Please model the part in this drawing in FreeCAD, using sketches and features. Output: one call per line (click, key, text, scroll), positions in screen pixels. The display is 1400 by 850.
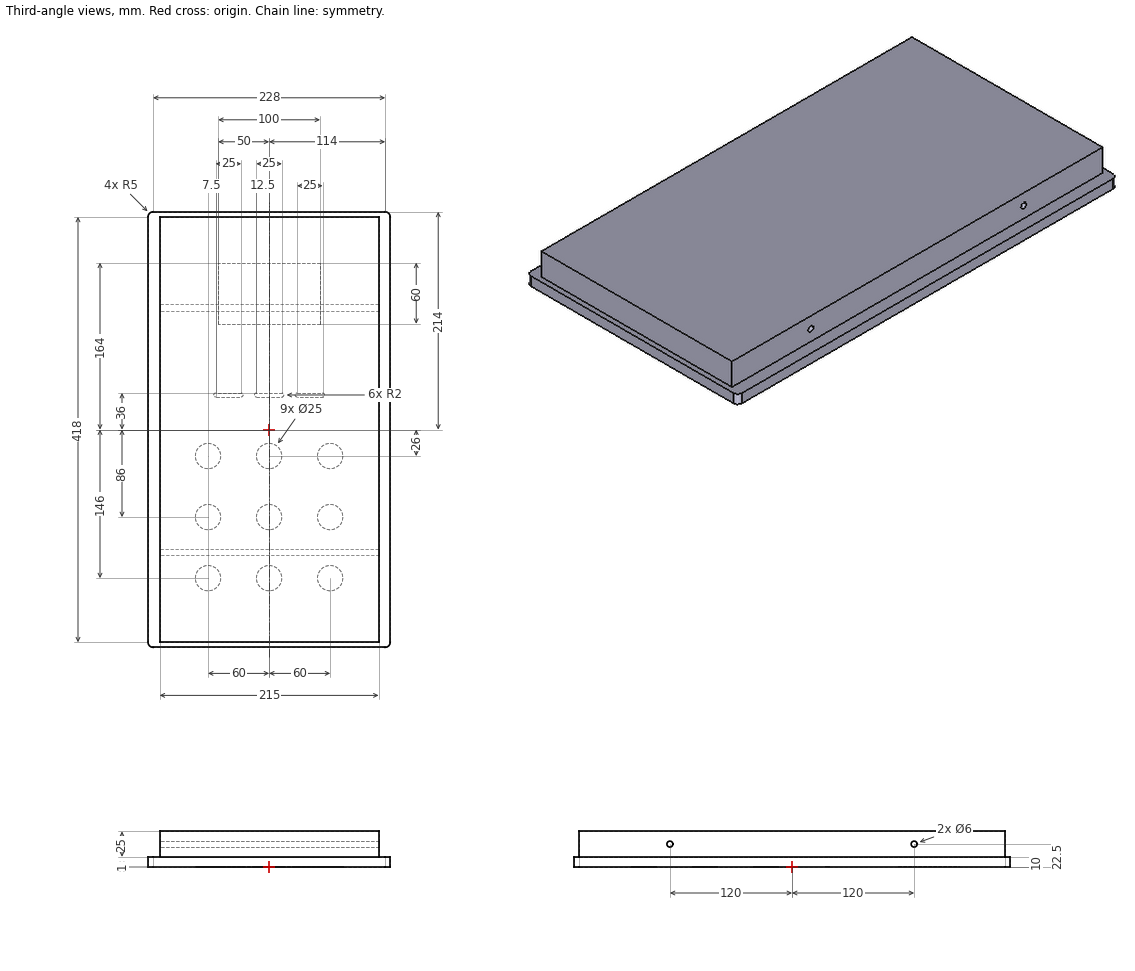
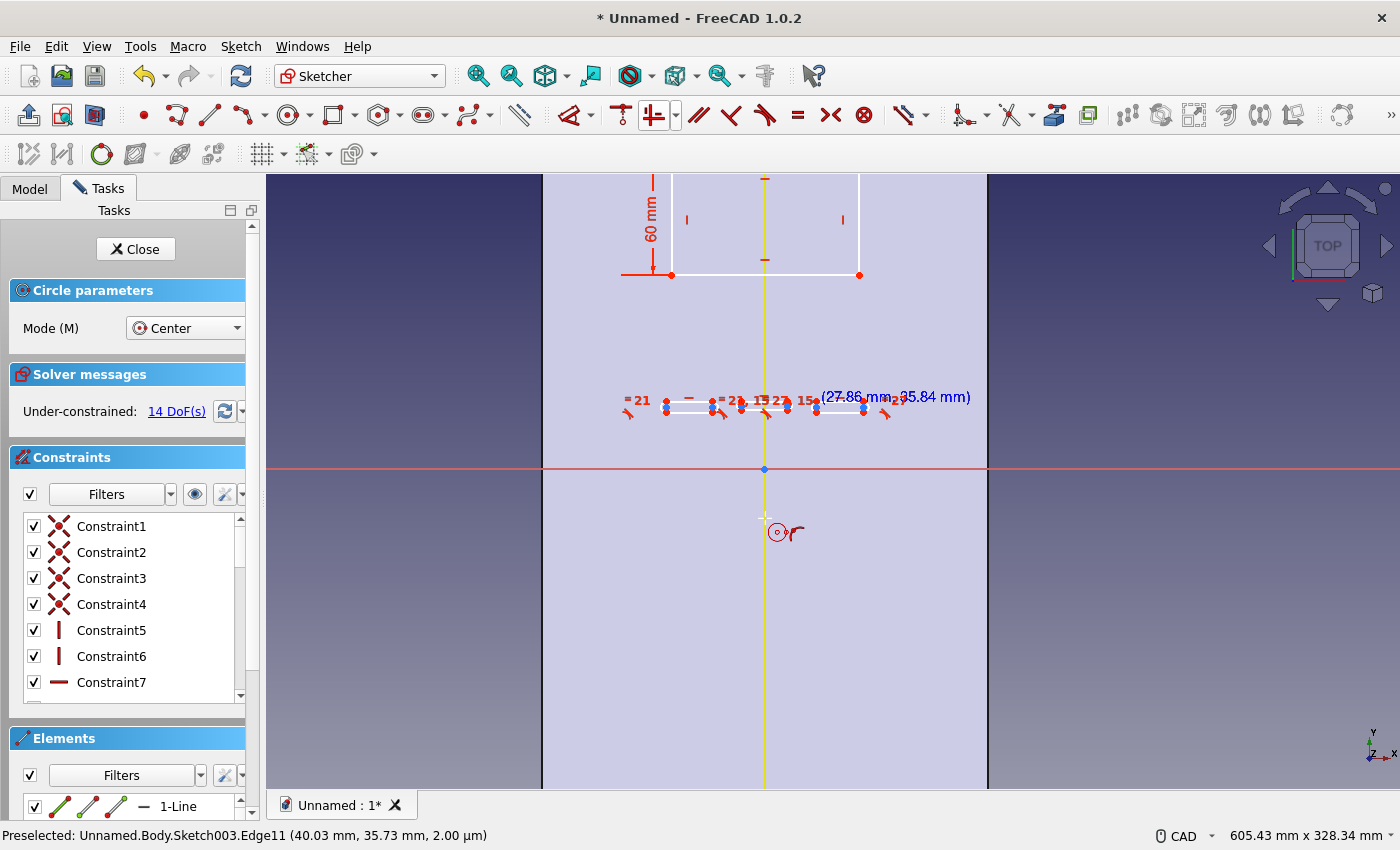
click(765, 518)
move(781, 501)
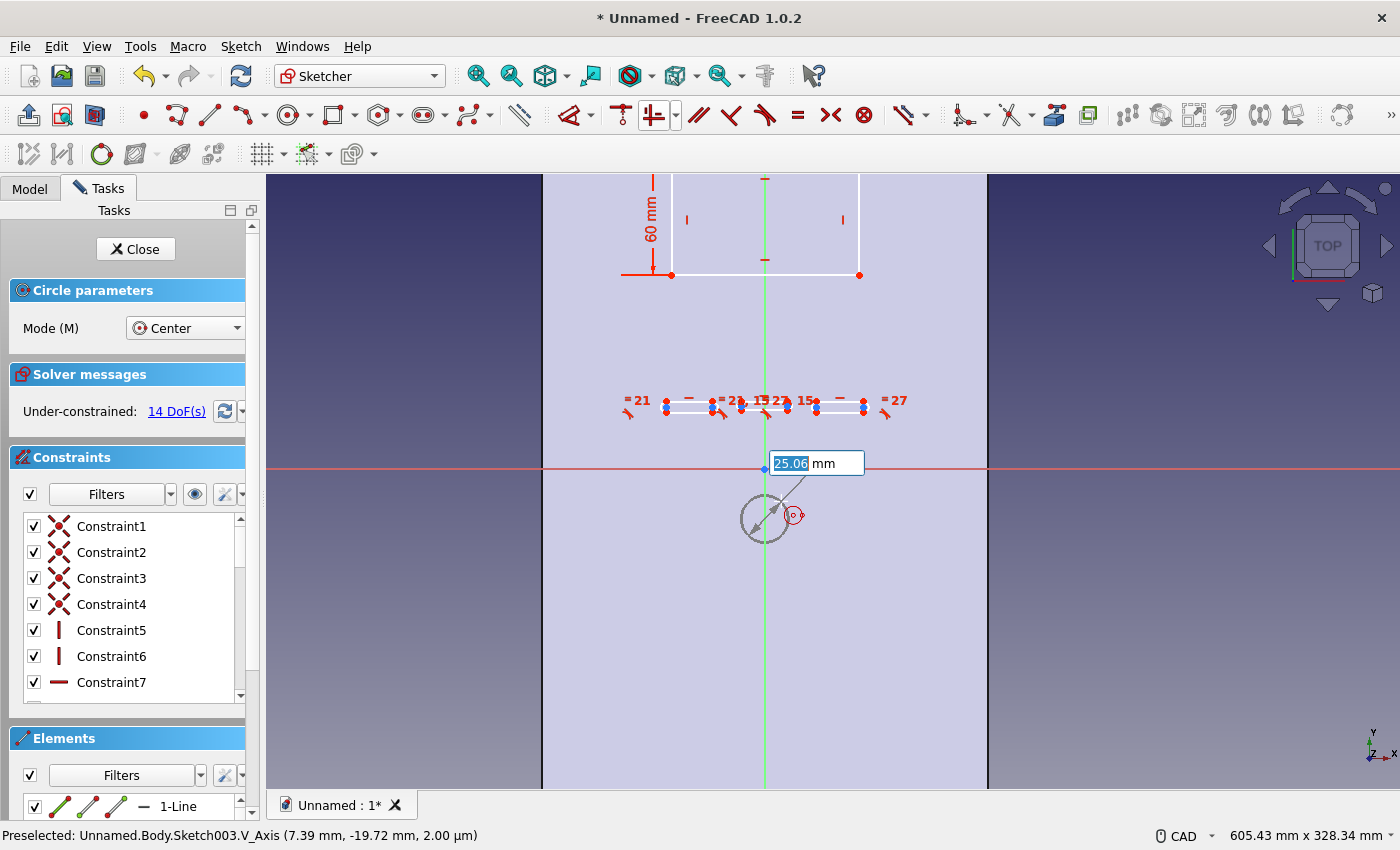
text(25)
key(Return)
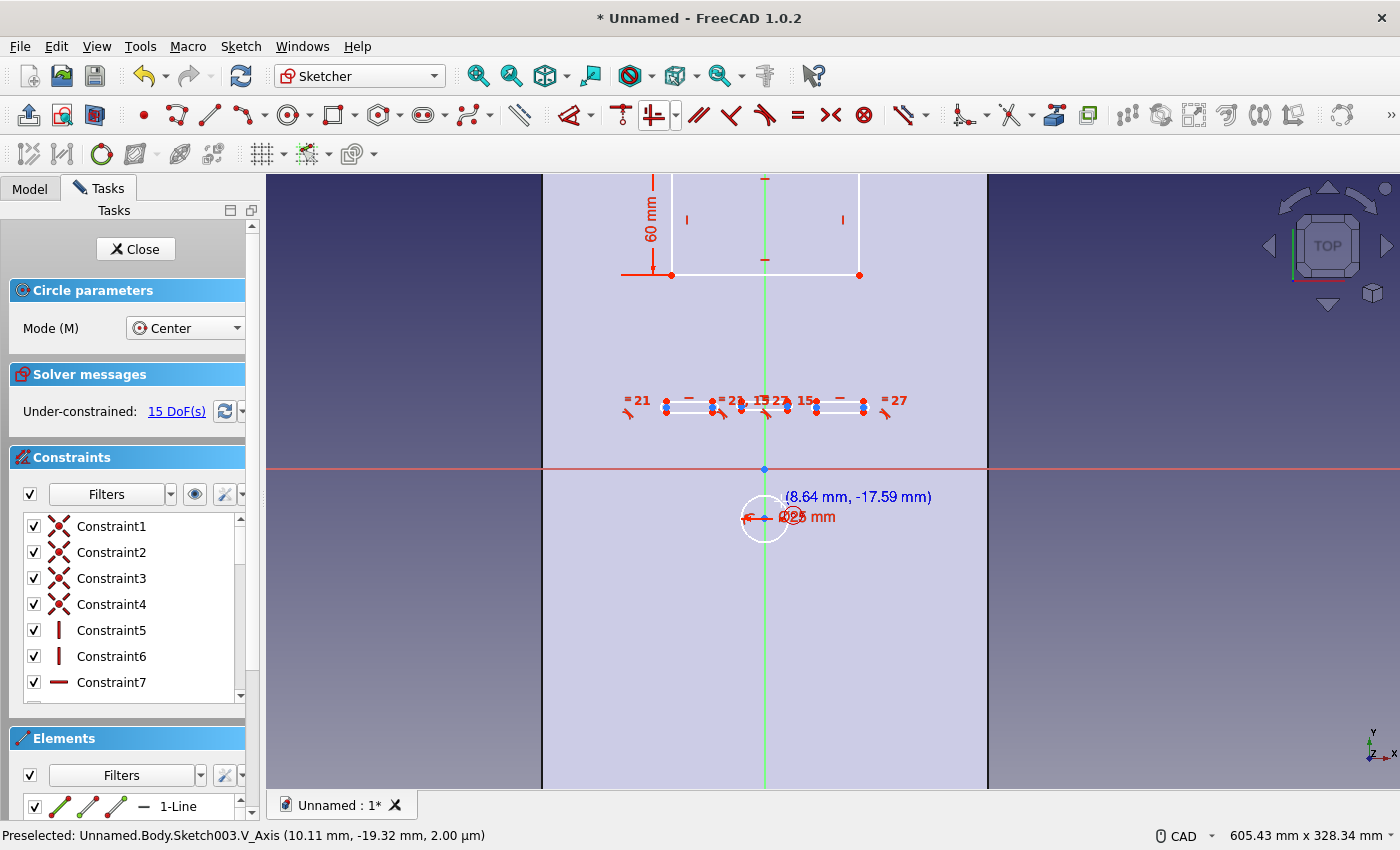
click(652, 518)
move(669, 501)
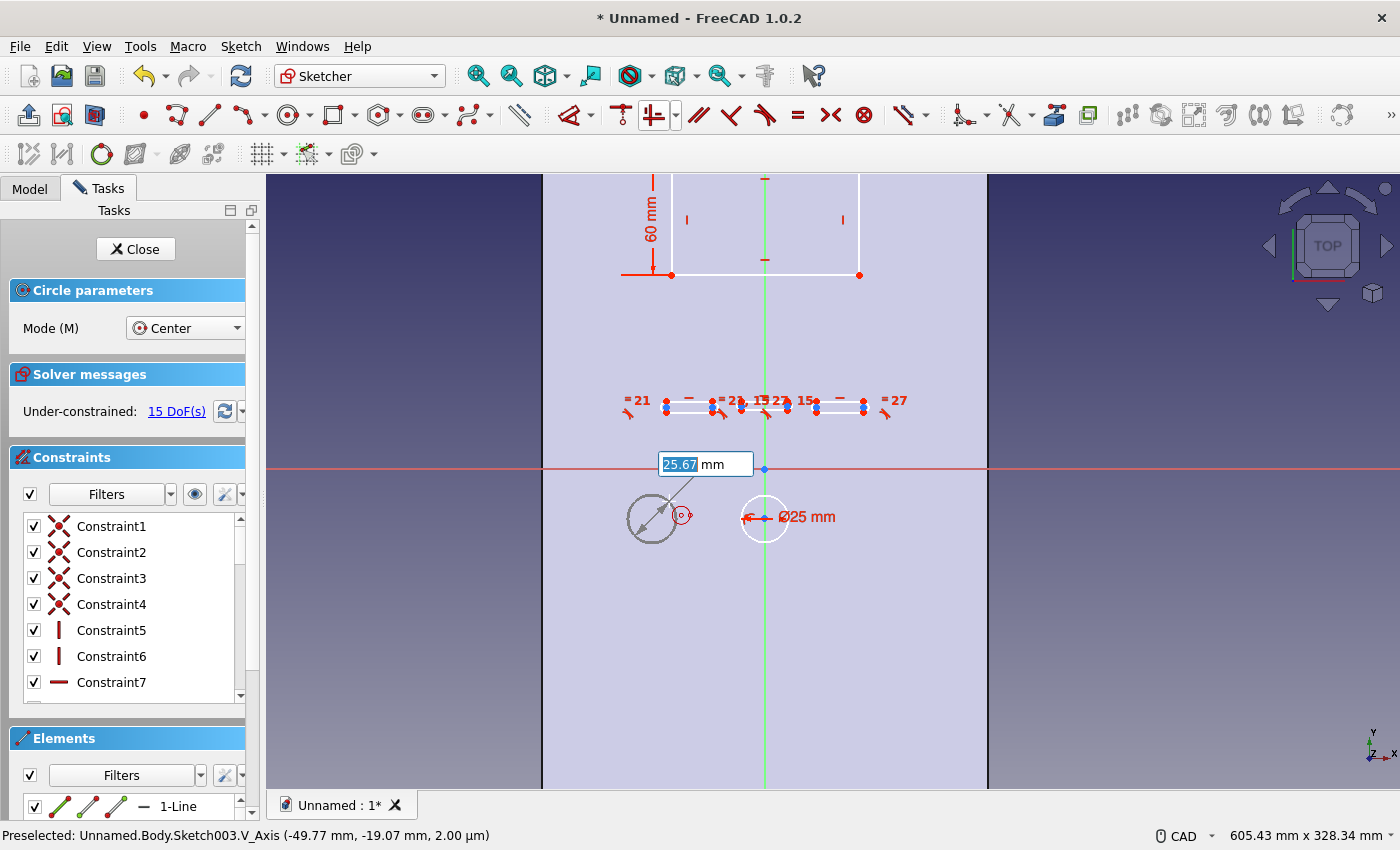
text(25)
key(Return)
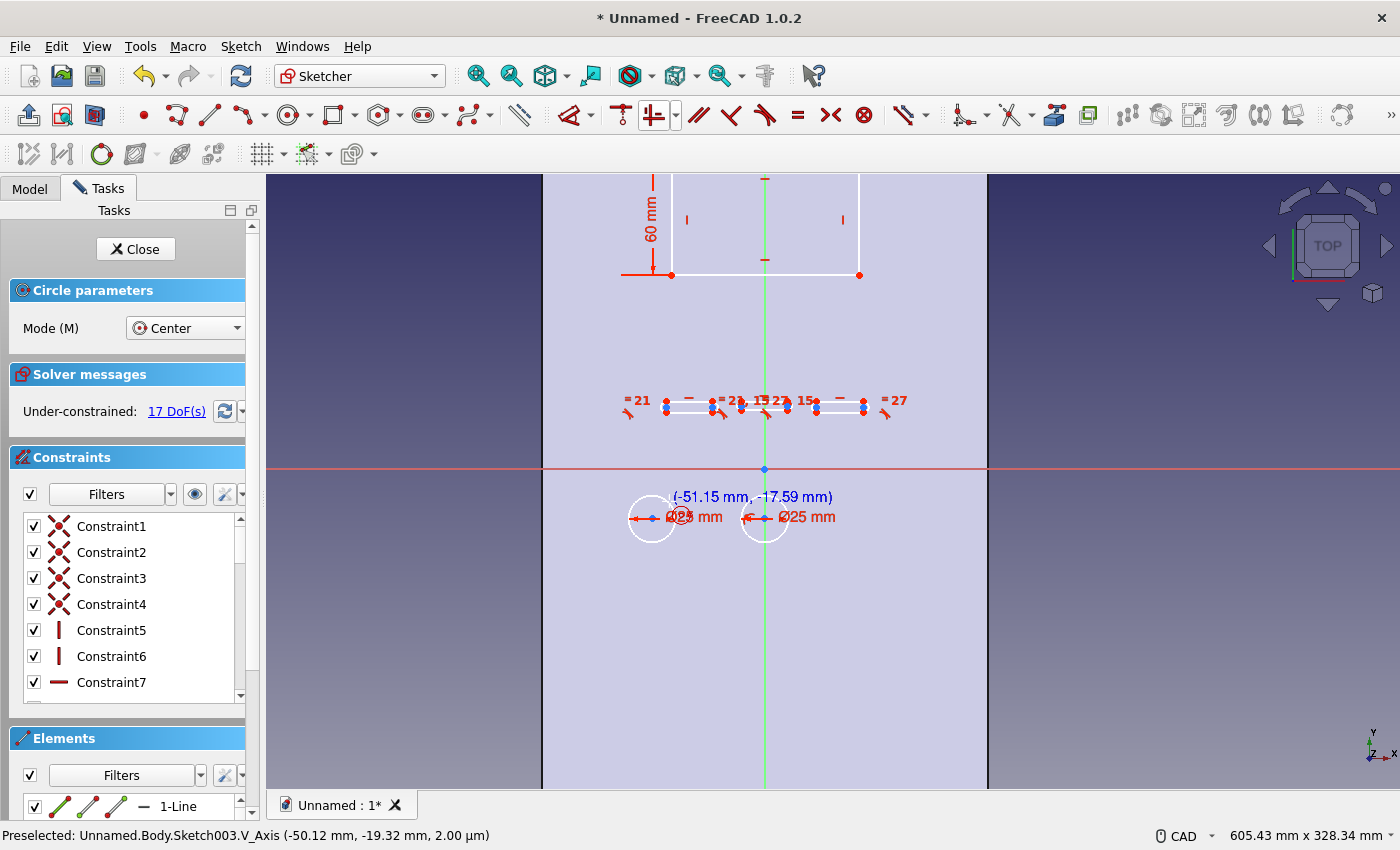
click(652, 630)
move(669, 614)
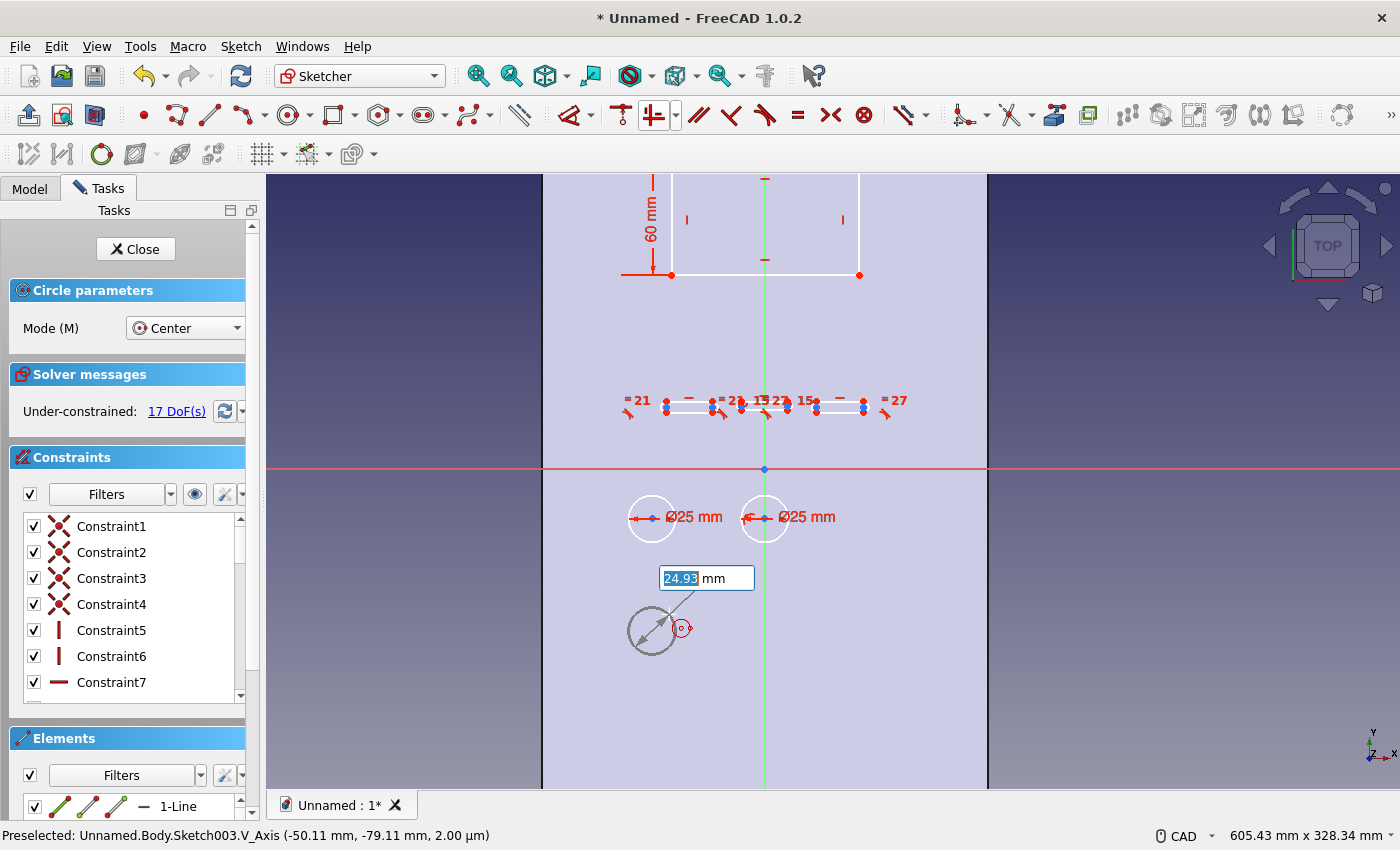
text(25)
key(Return)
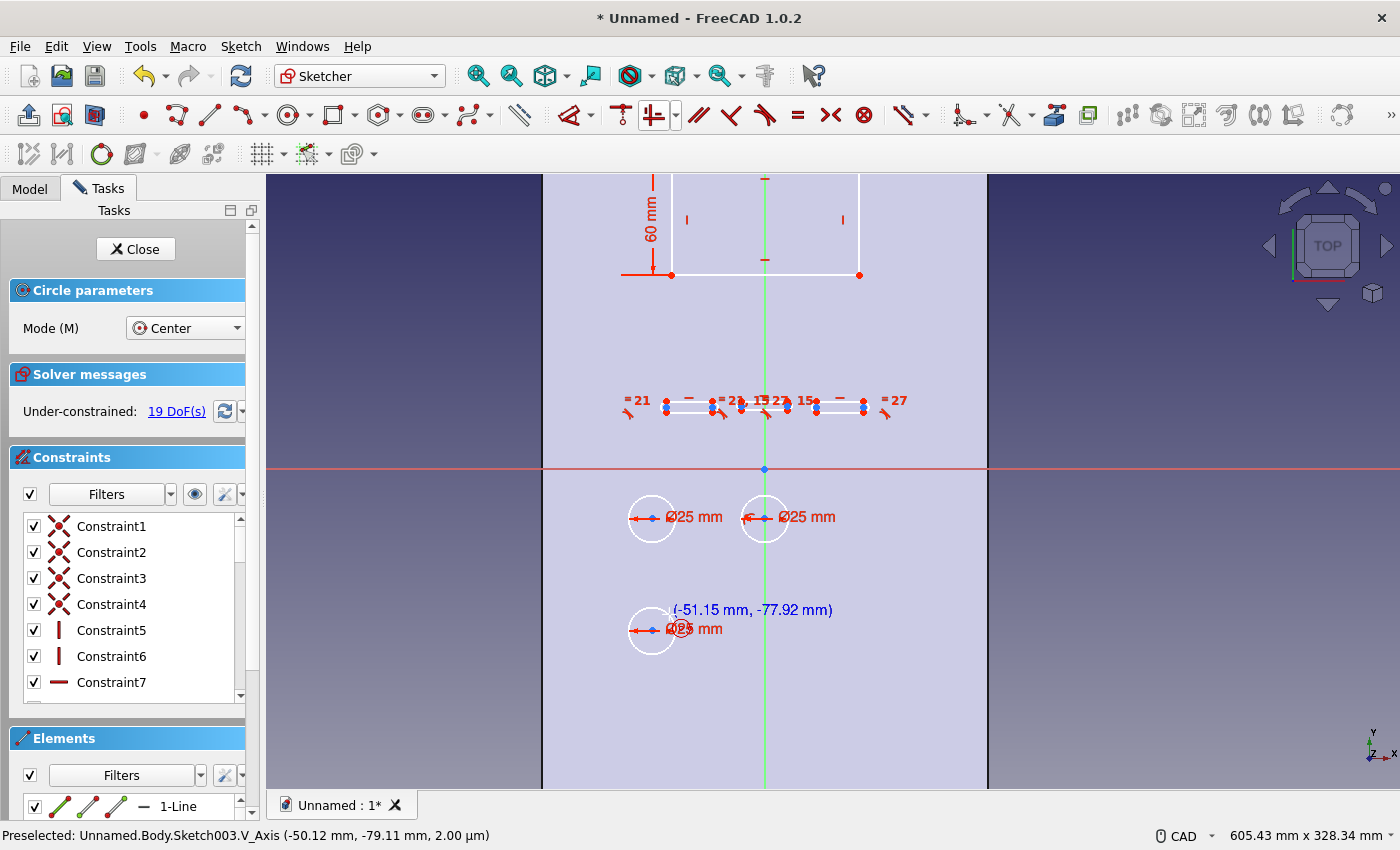
click(652, 743)
move(669, 726)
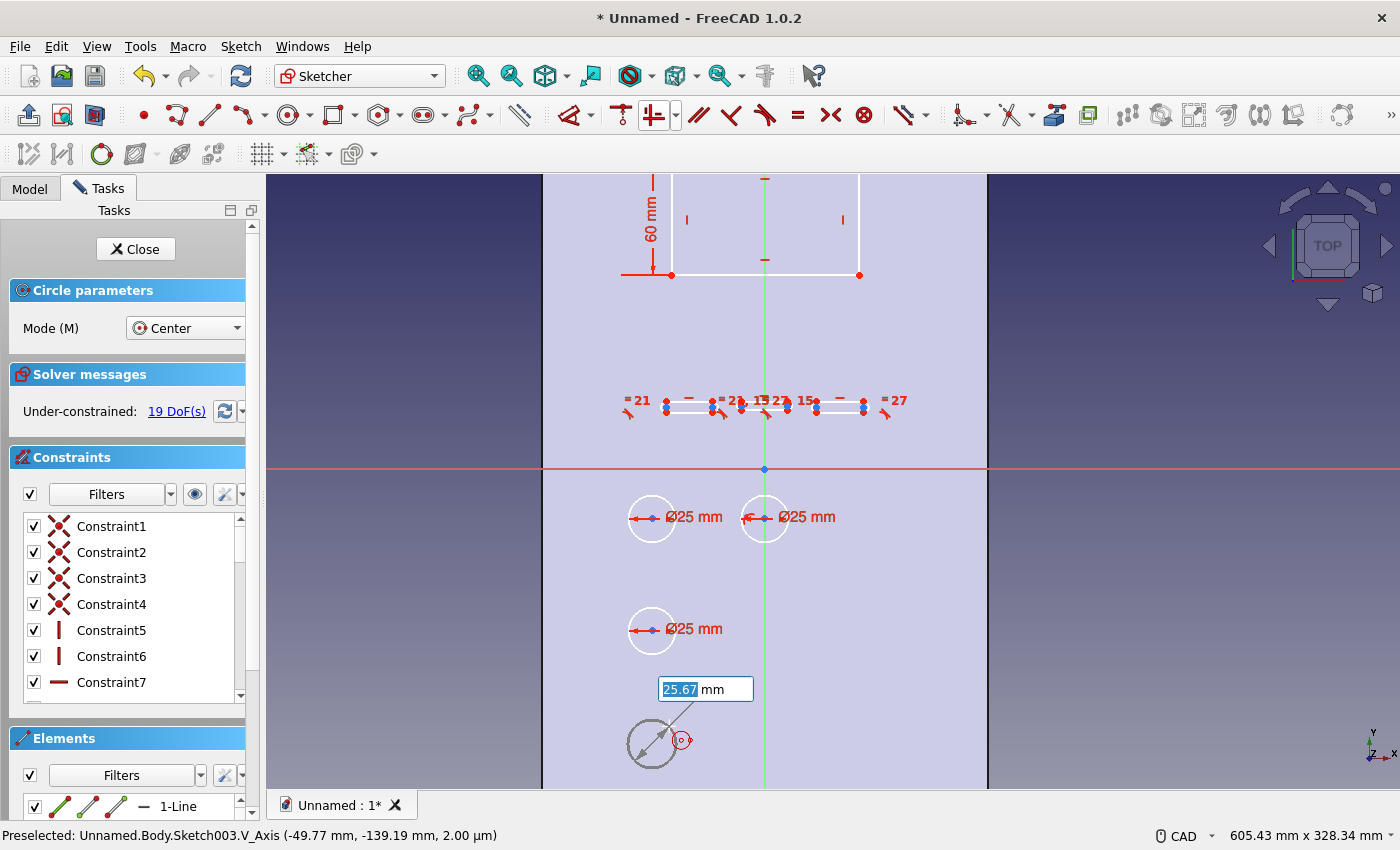
text(25)
key(Return)